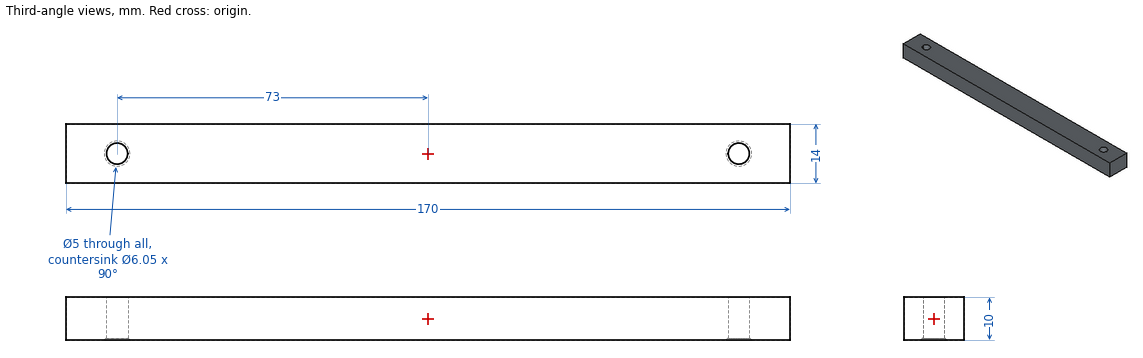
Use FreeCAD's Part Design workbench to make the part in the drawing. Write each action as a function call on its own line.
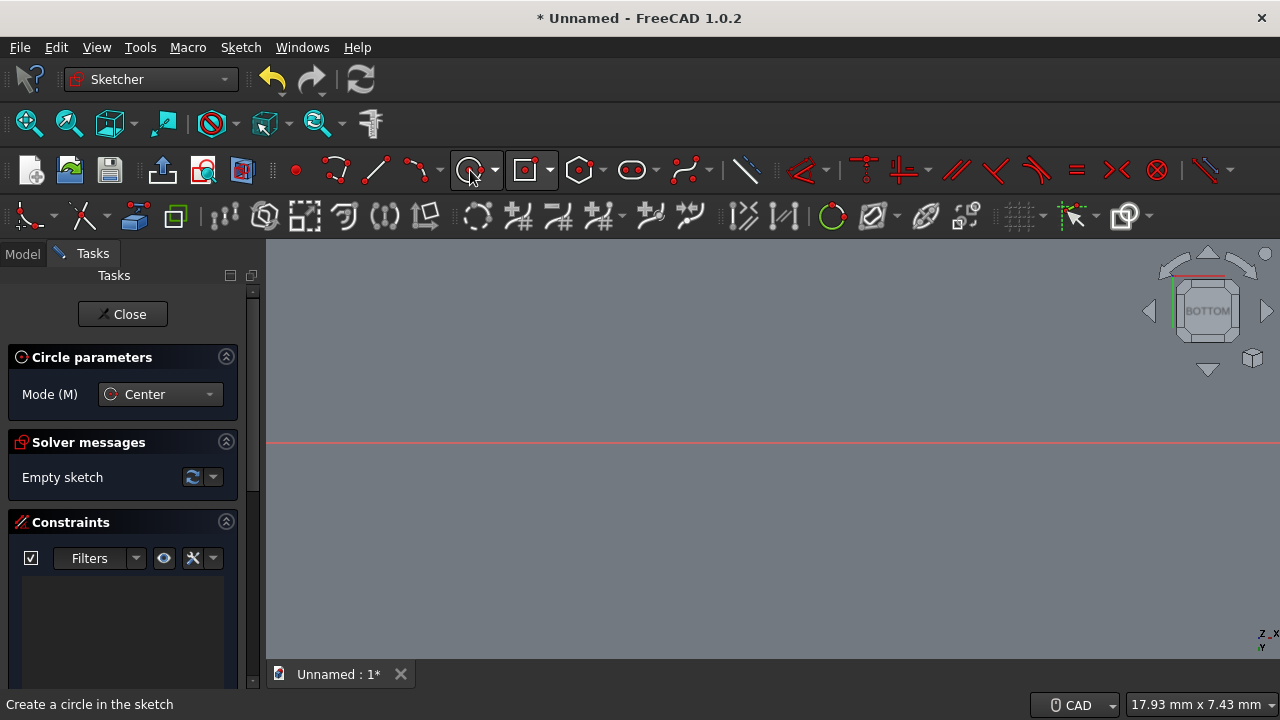
click(706, 443)
click(806, 343)
key(Escape)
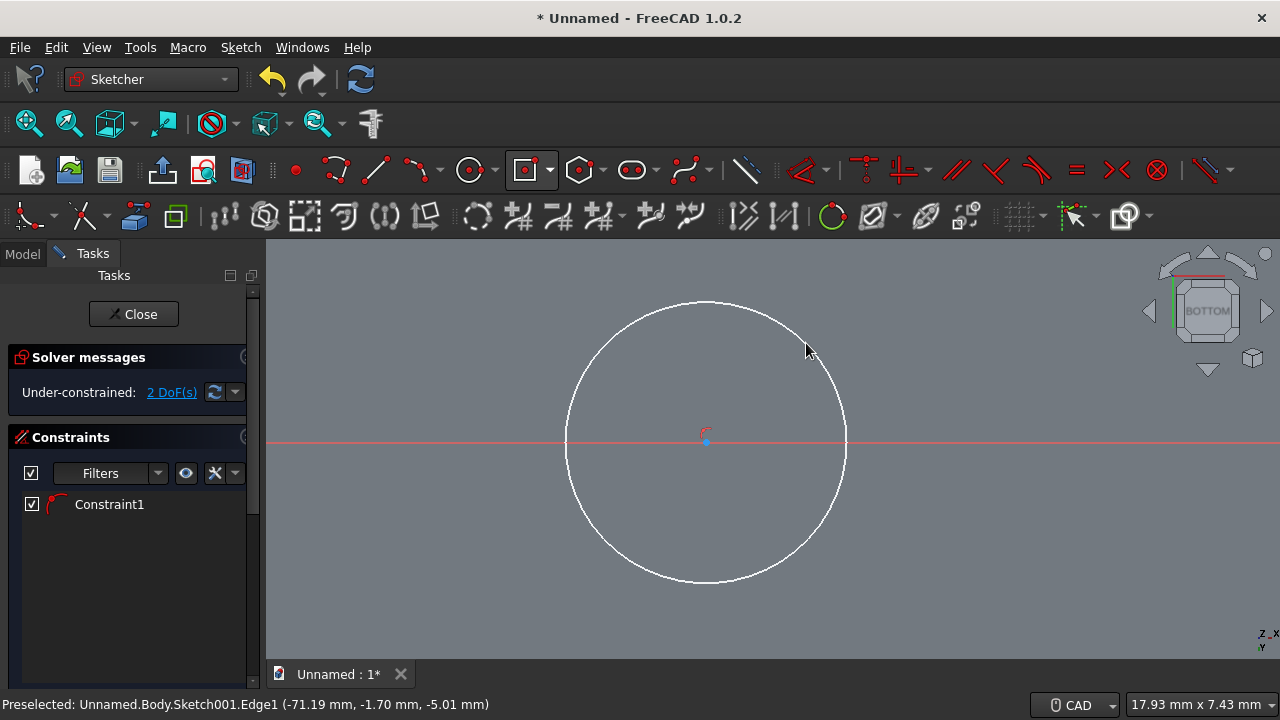
key(d)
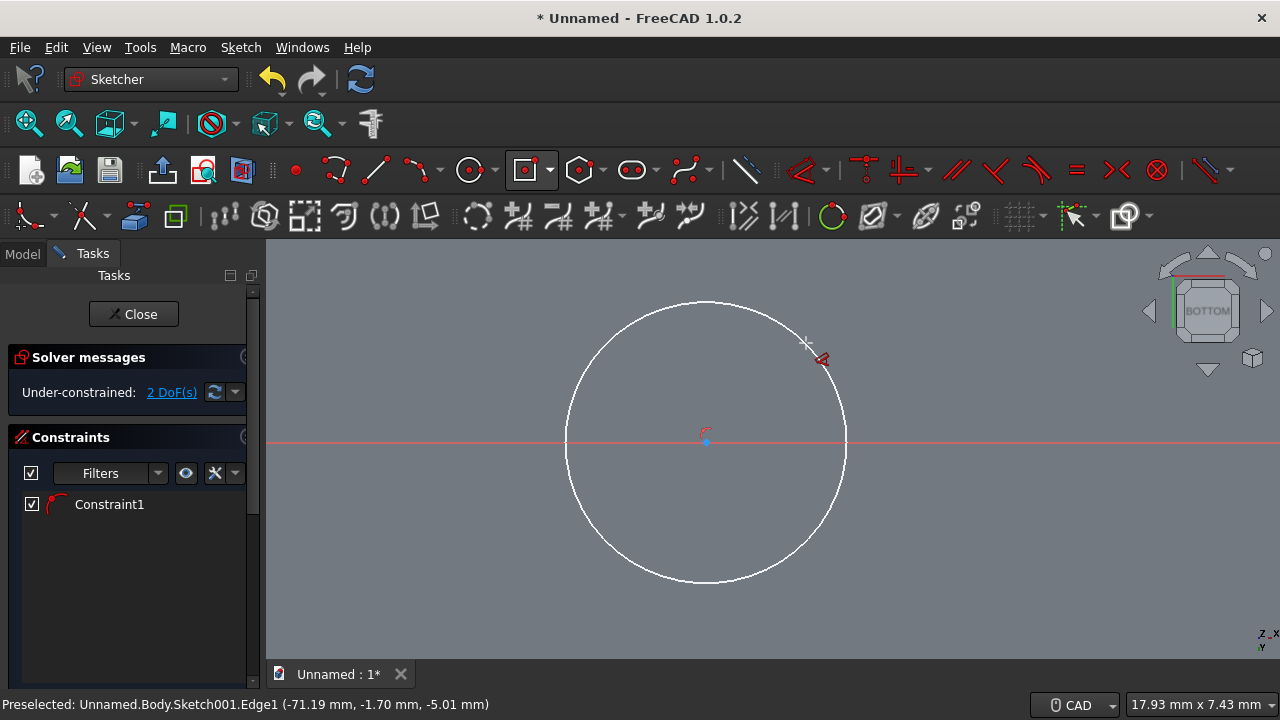
click(805, 343)
click(828, 320)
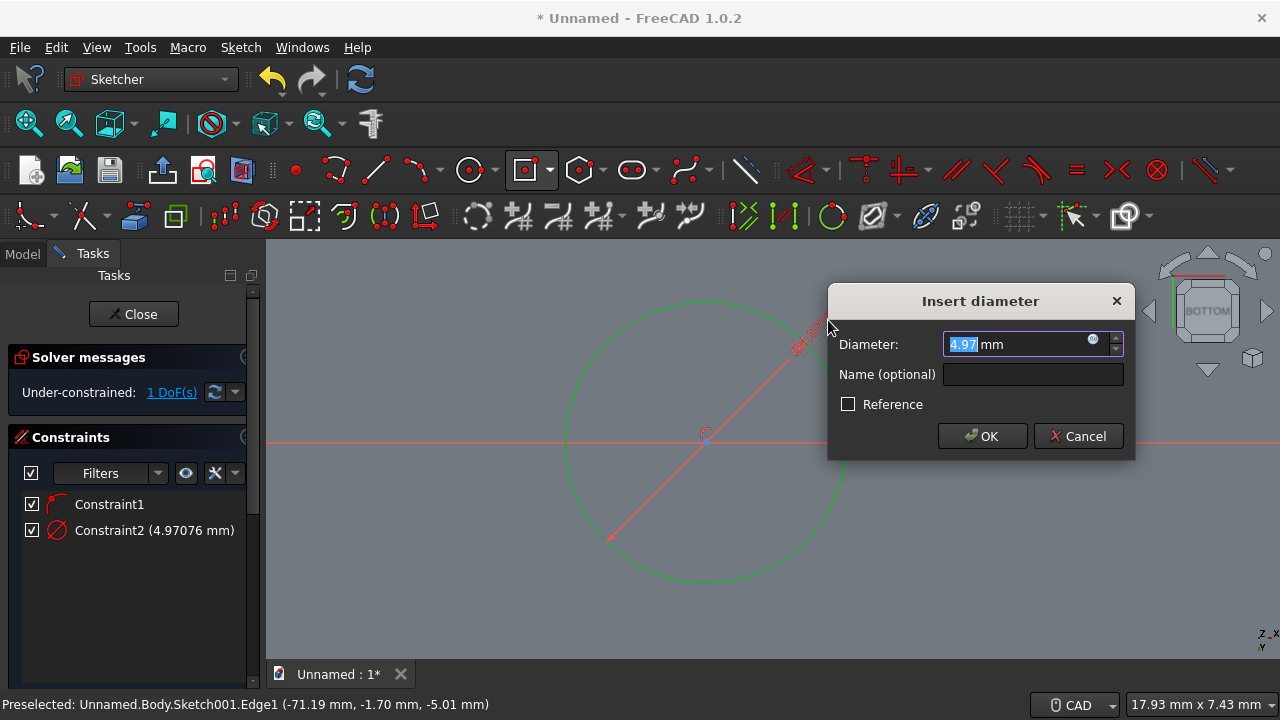
text(5)
key(Return)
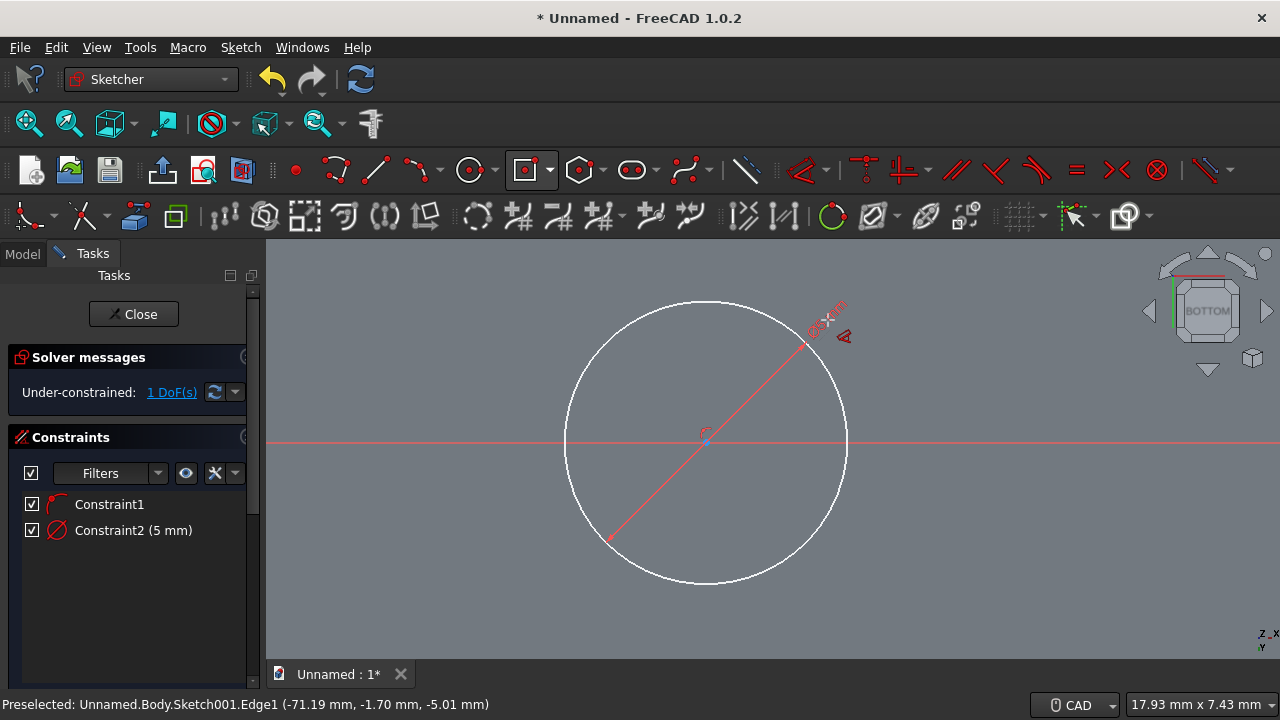
click(706, 443)
click(911, 477)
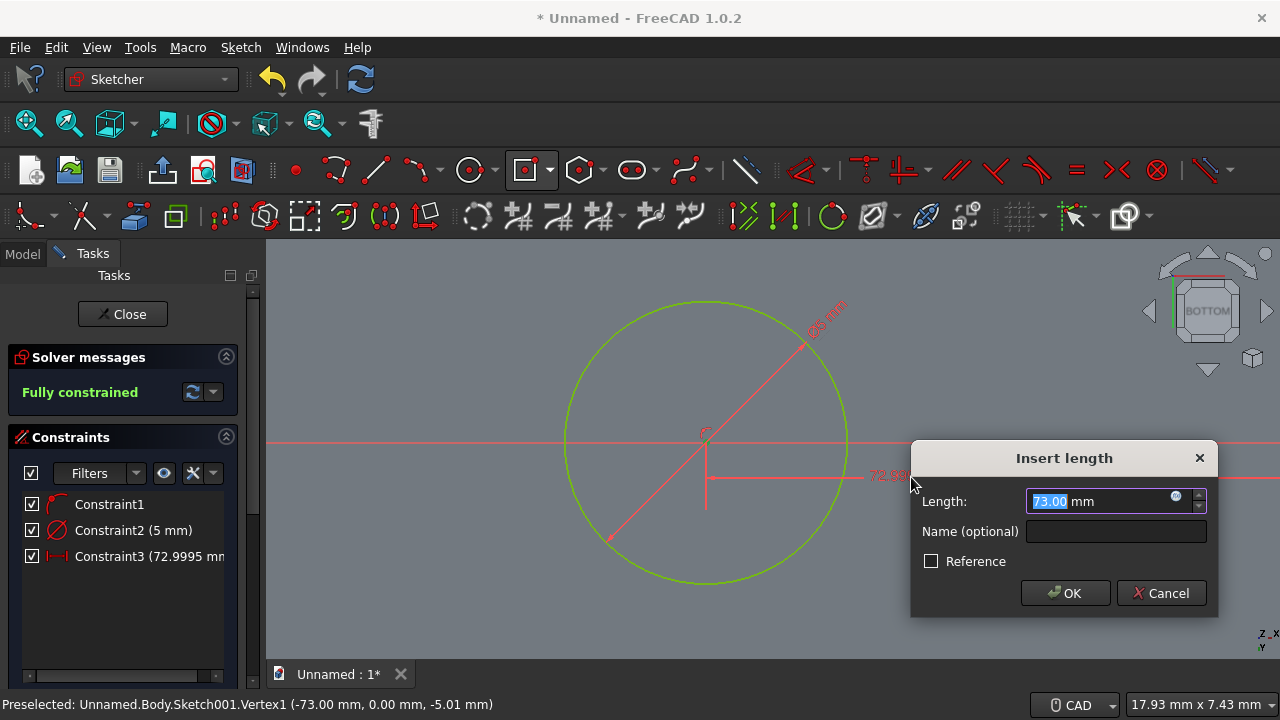
text(73)
key(Return)
key(Escape)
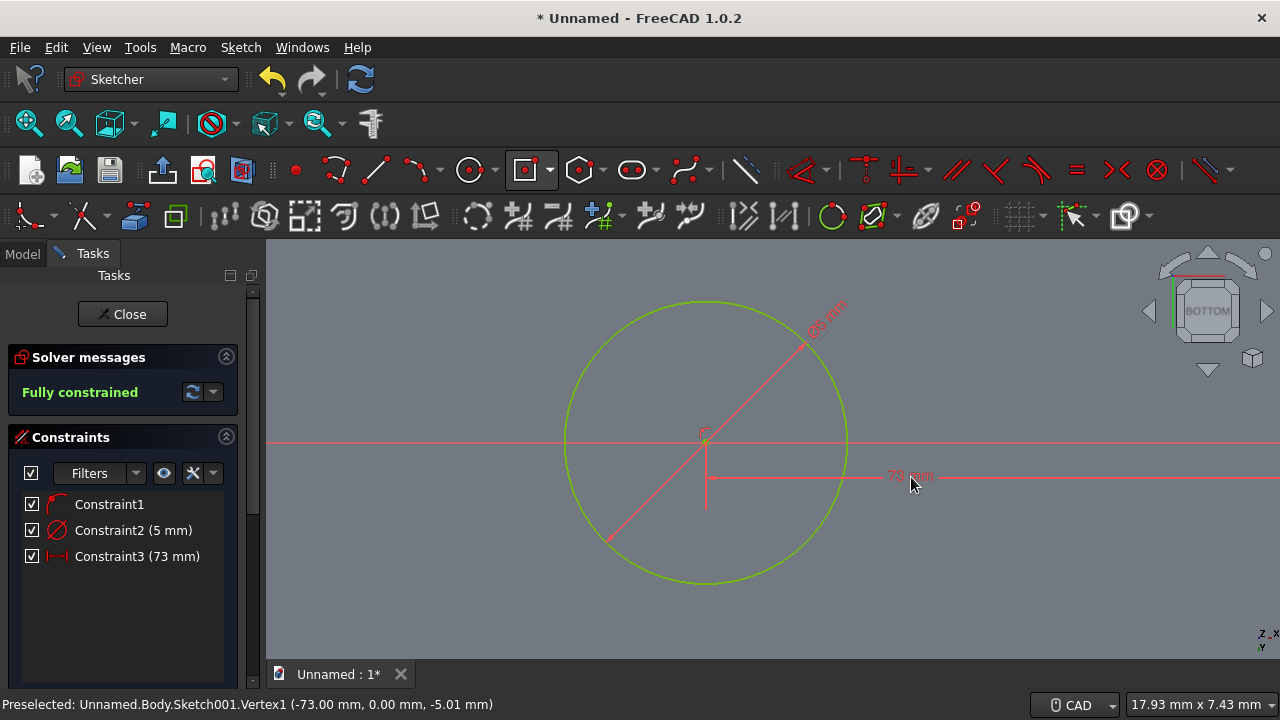
click(123, 314)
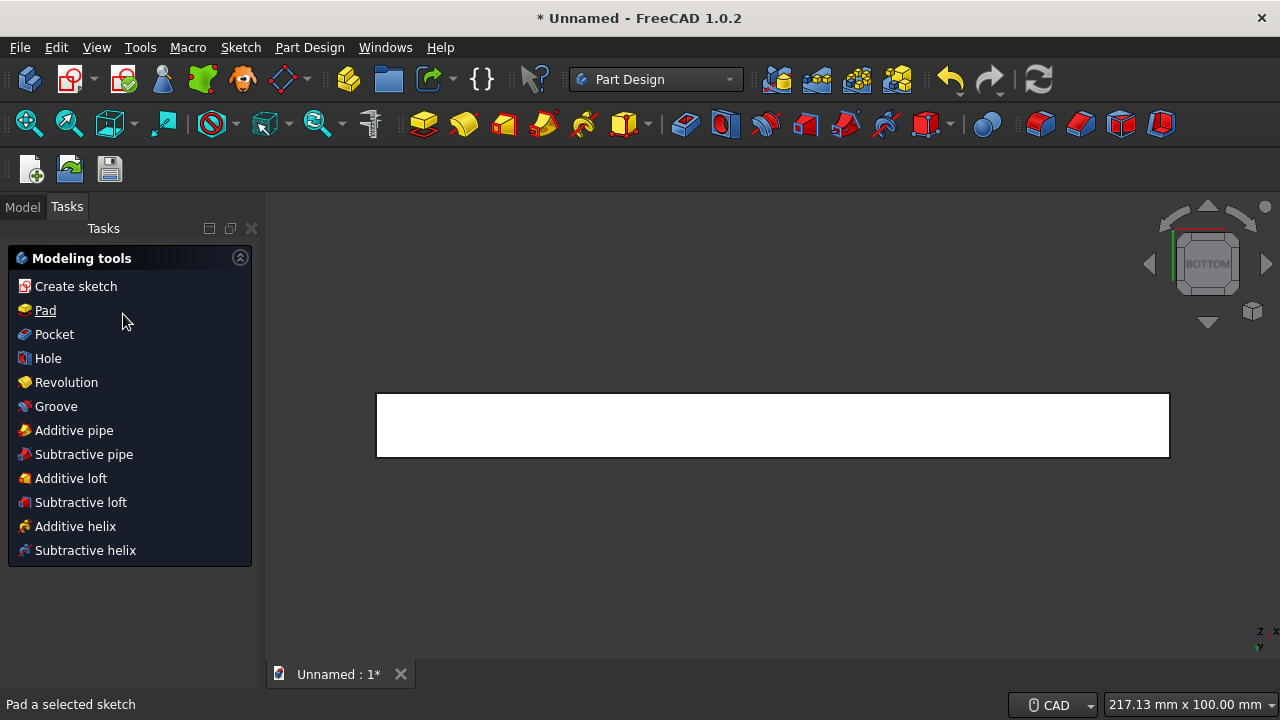
click(726, 124)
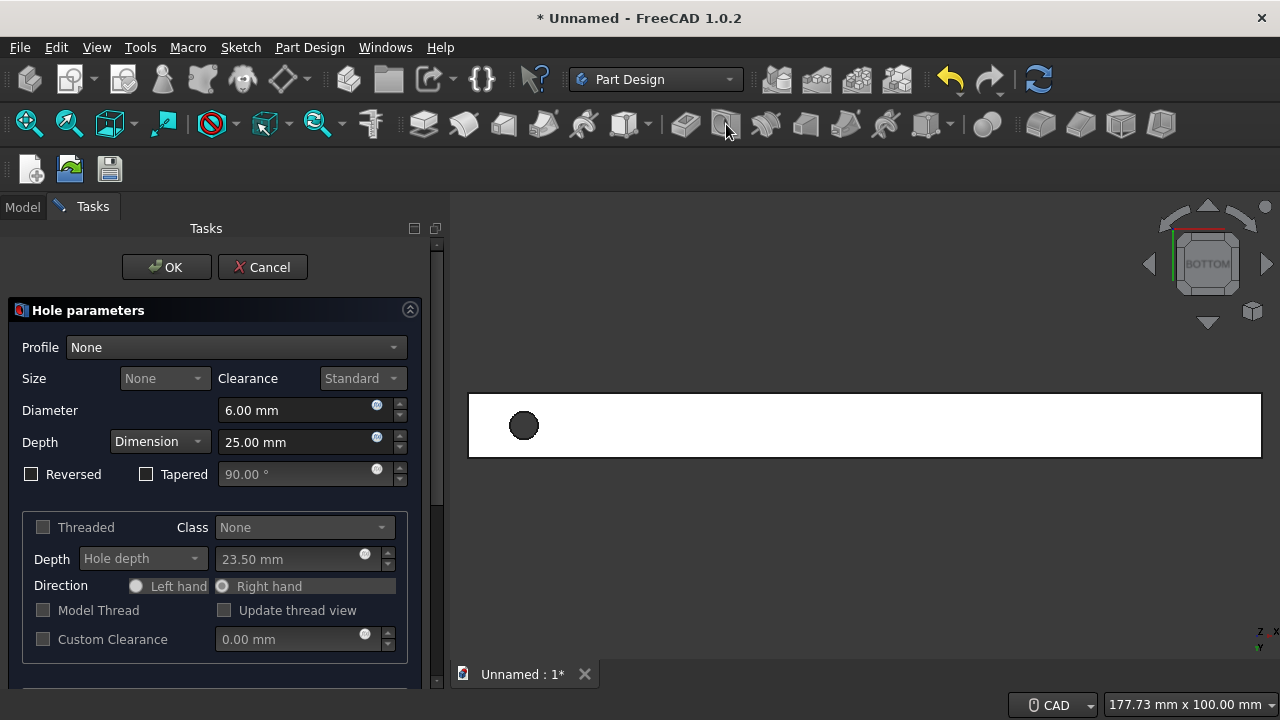
triple_click(305, 410)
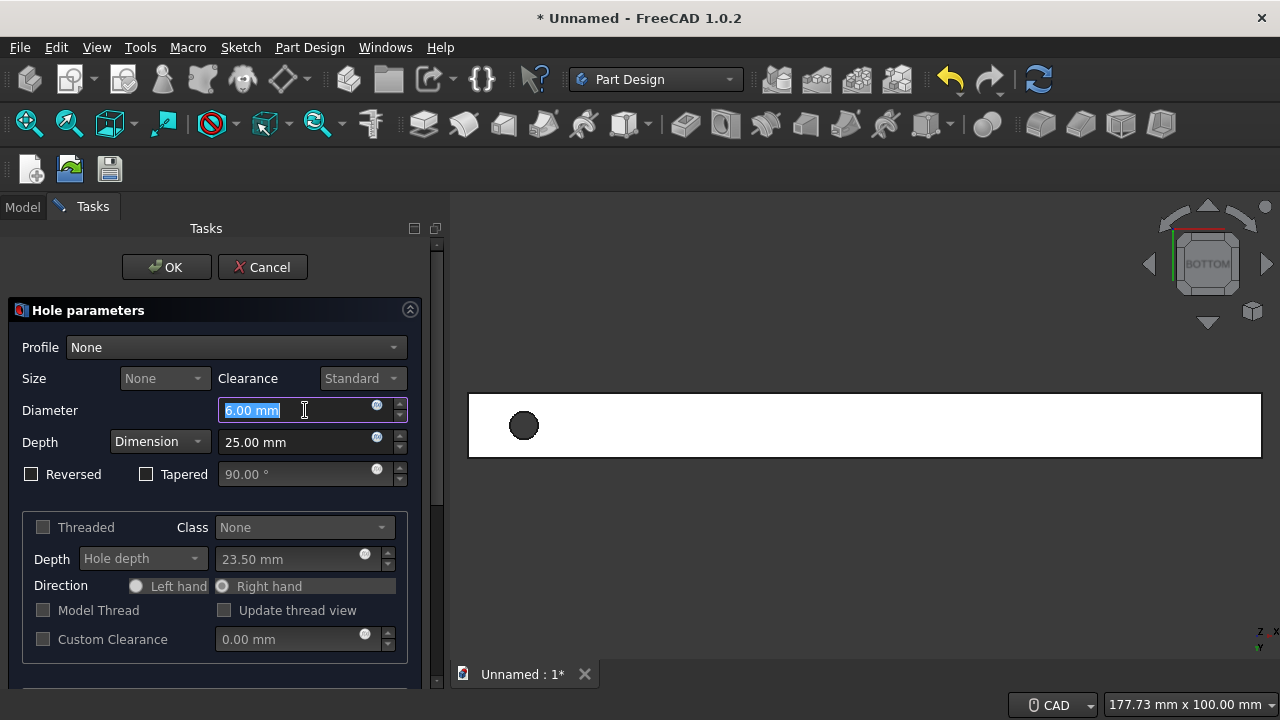
text(5)
key(Tab)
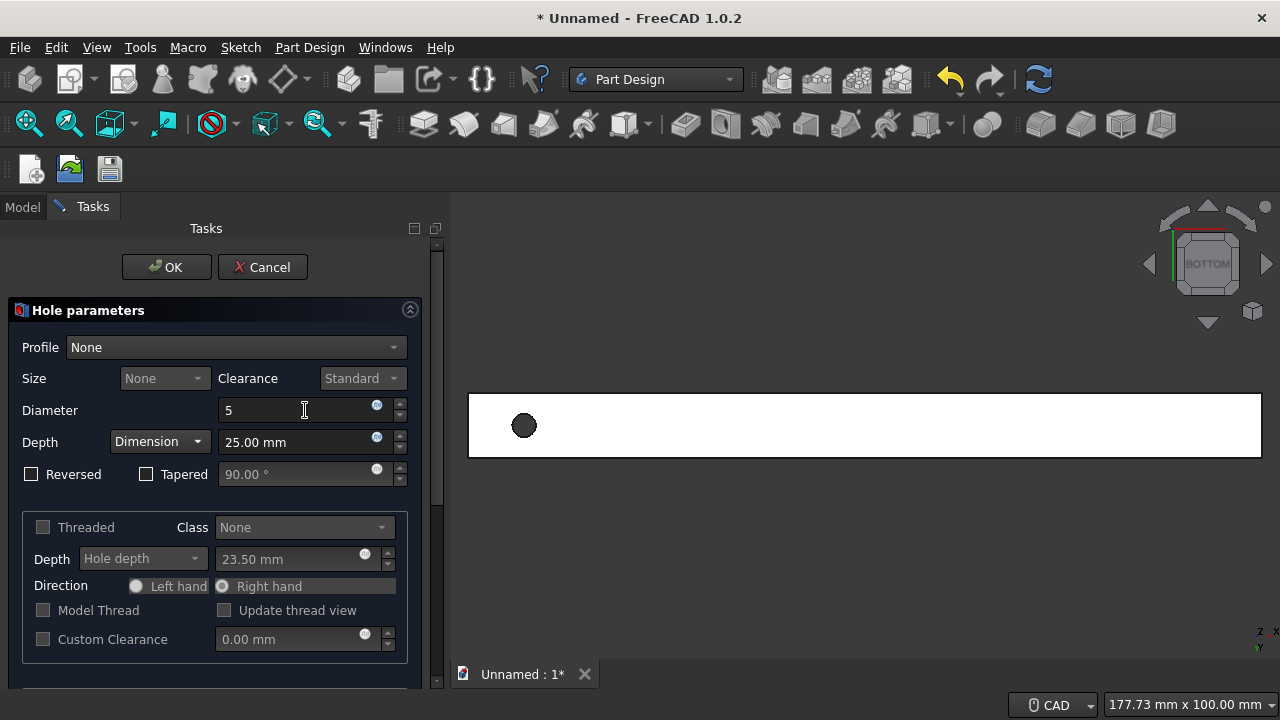
click(161, 442)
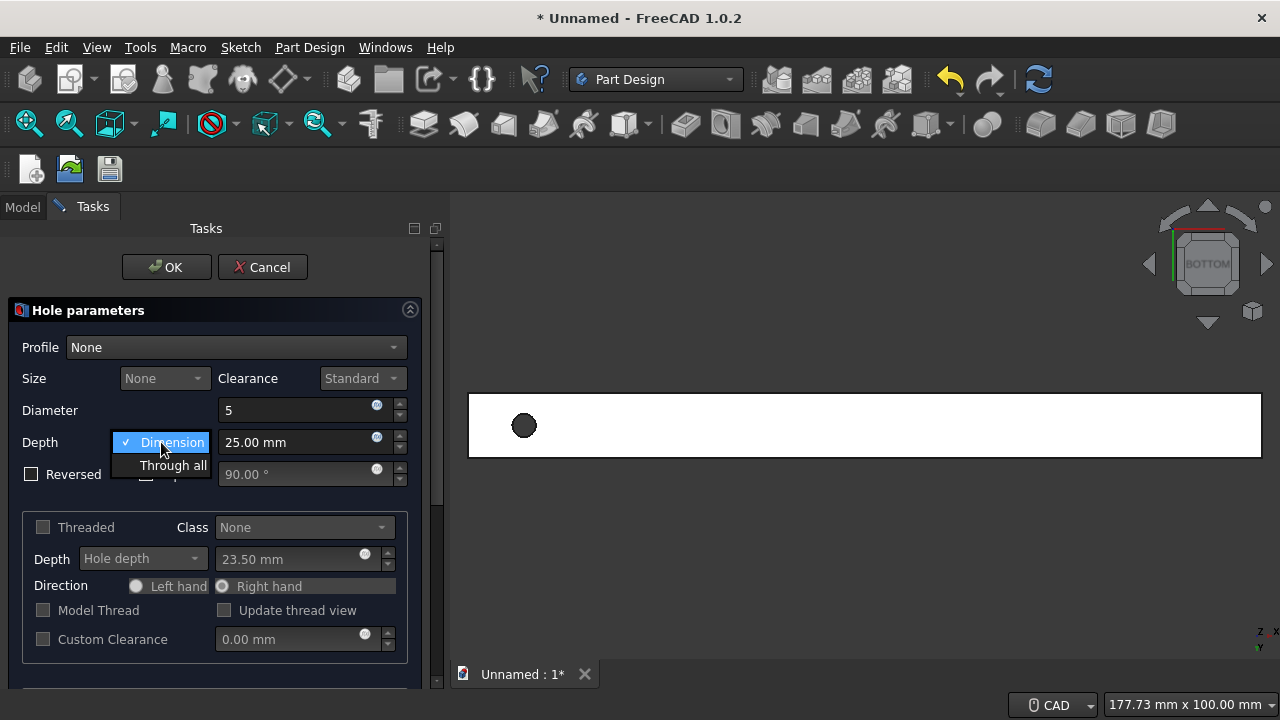
click(160, 466)